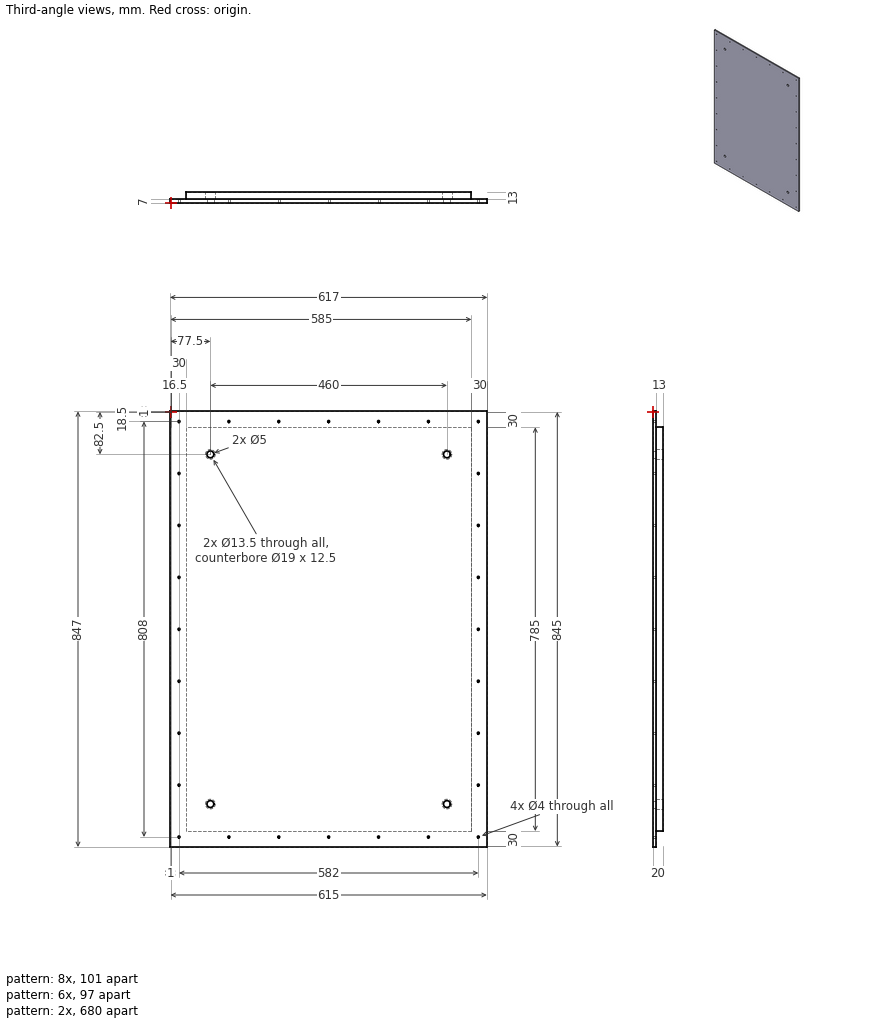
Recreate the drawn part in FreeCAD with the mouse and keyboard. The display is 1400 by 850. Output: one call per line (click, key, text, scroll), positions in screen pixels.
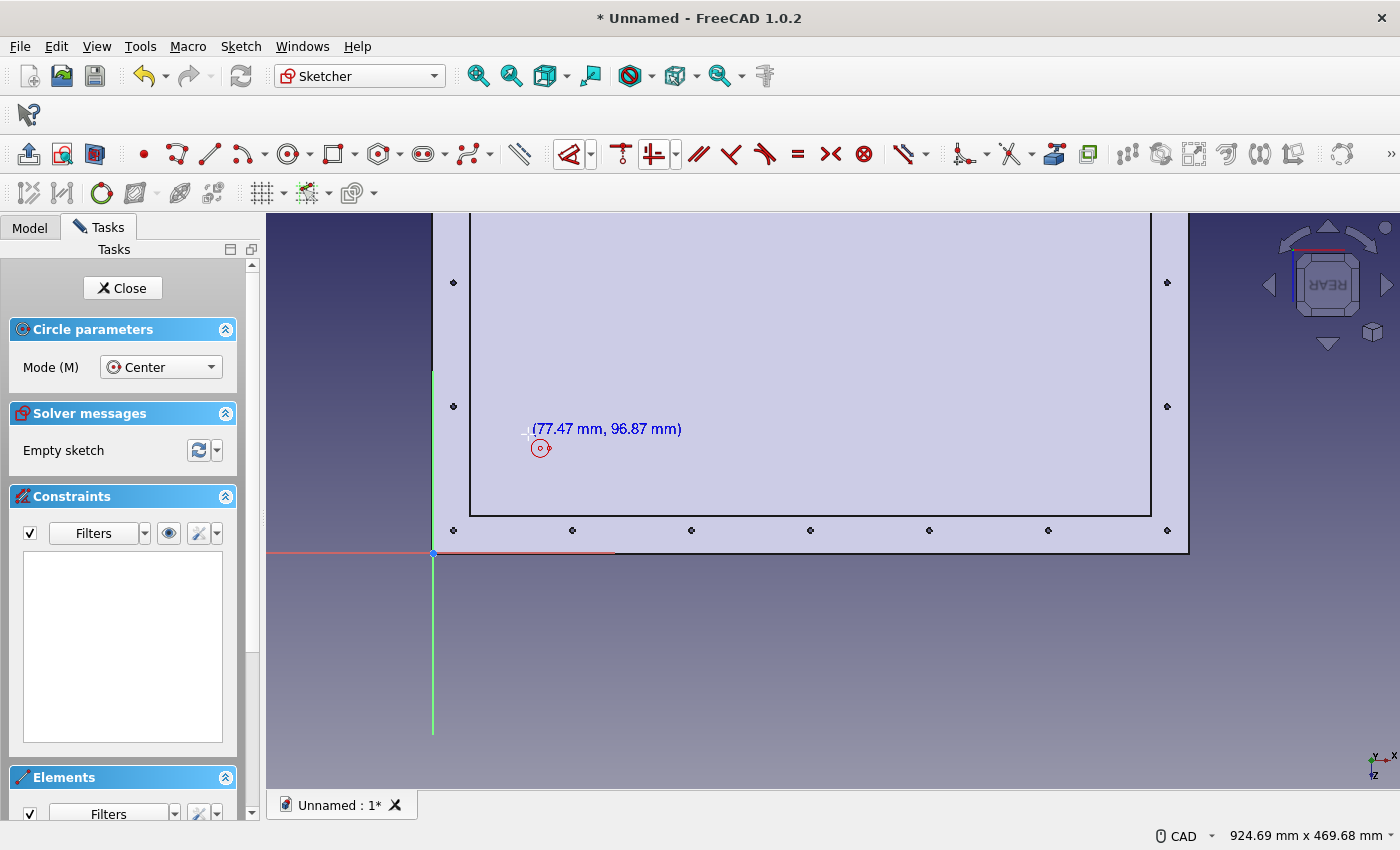
click(528, 452)
move(530, 450)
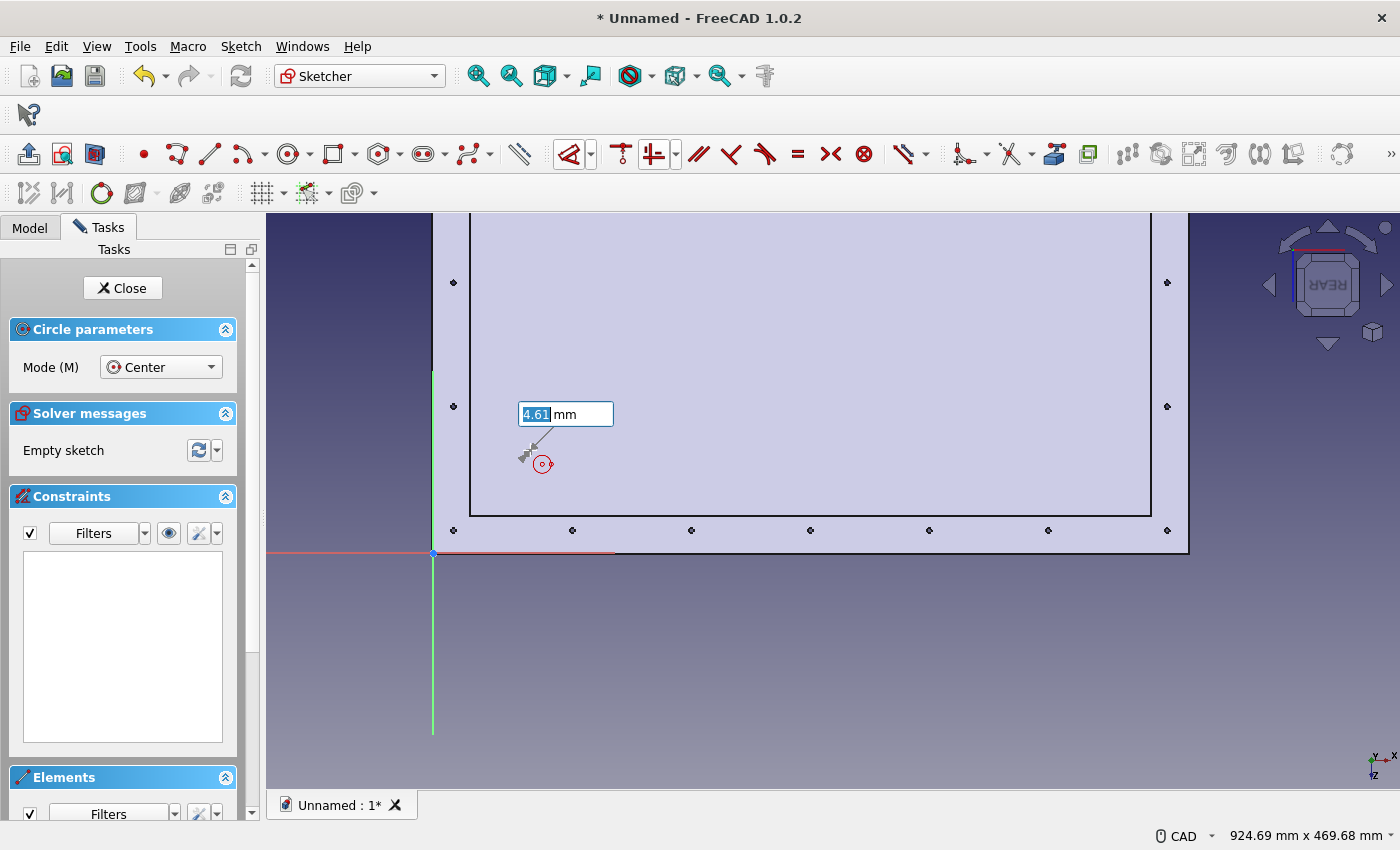
text(5)
key(Return)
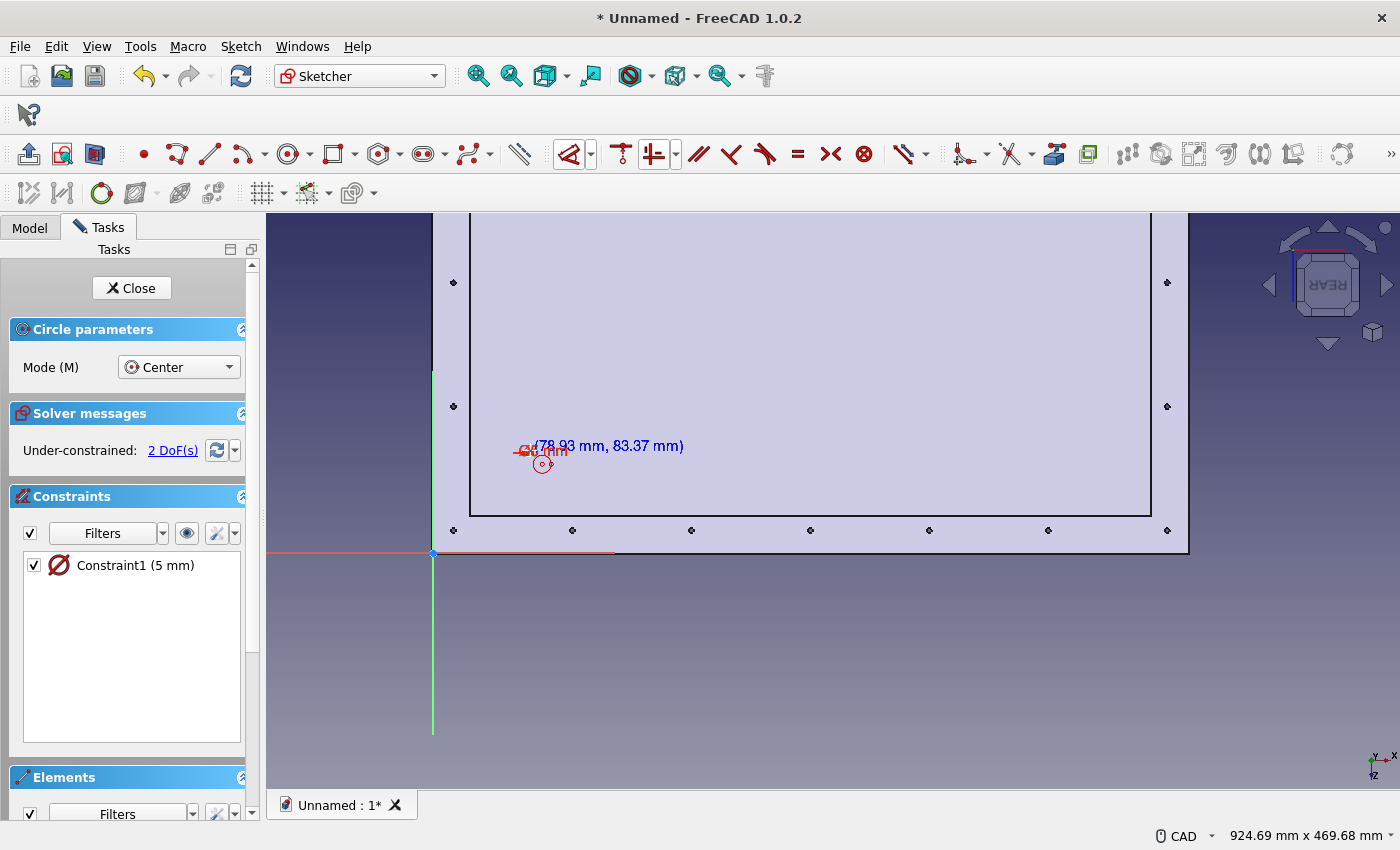
scroll(1092, 452, up, 11)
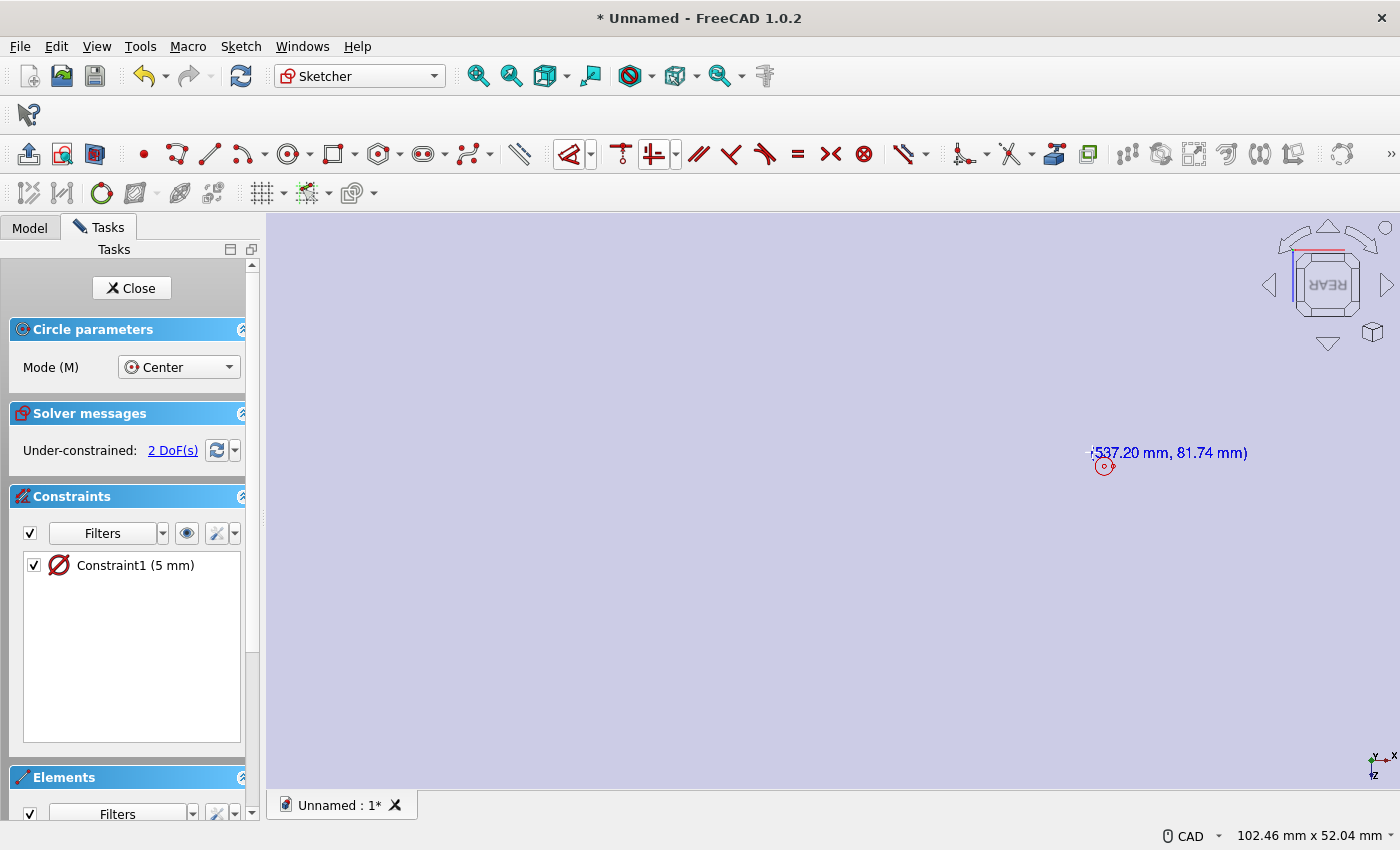
scroll(1093, 452, down, 11)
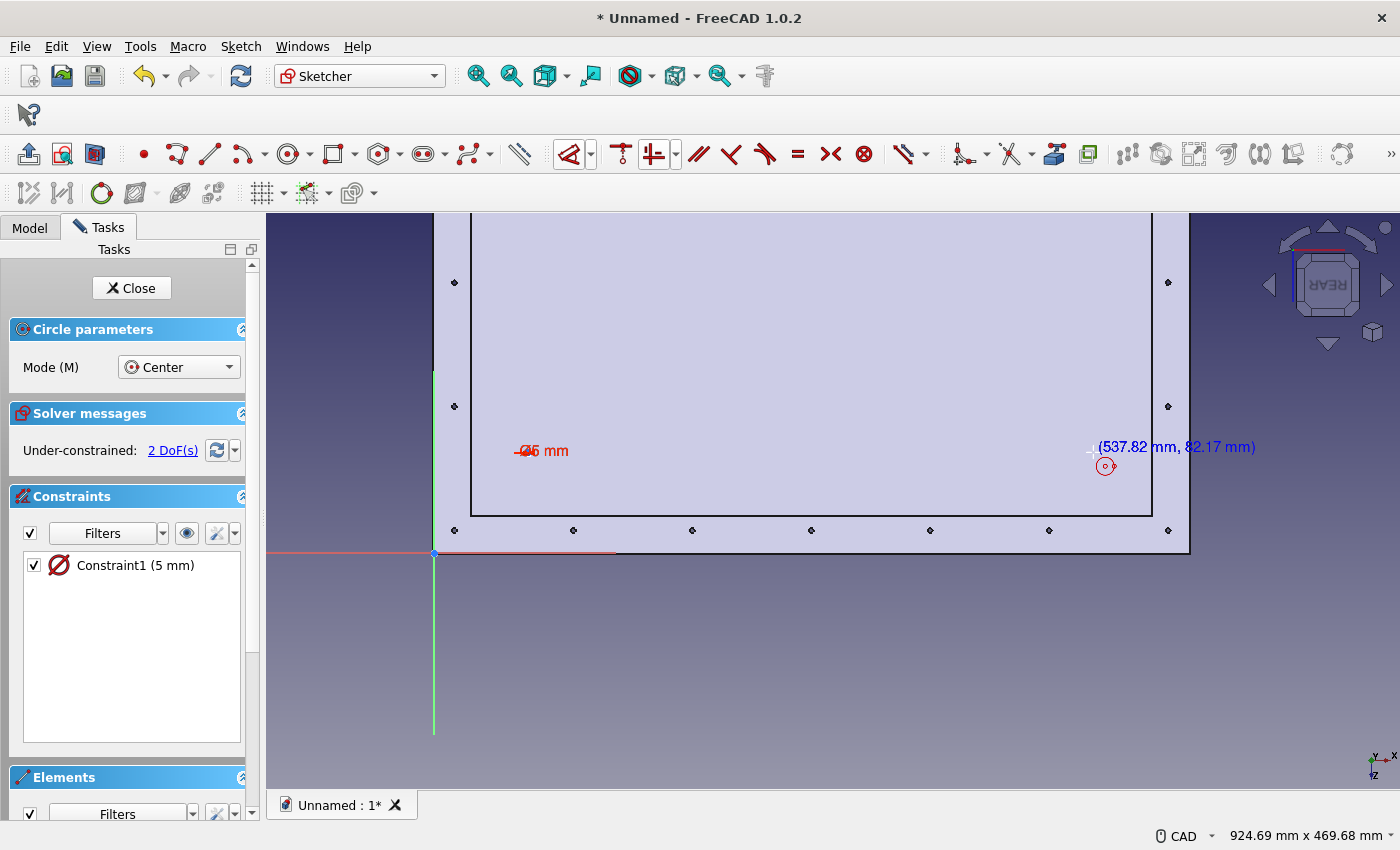
click(1093, 452)
move(1095, 450)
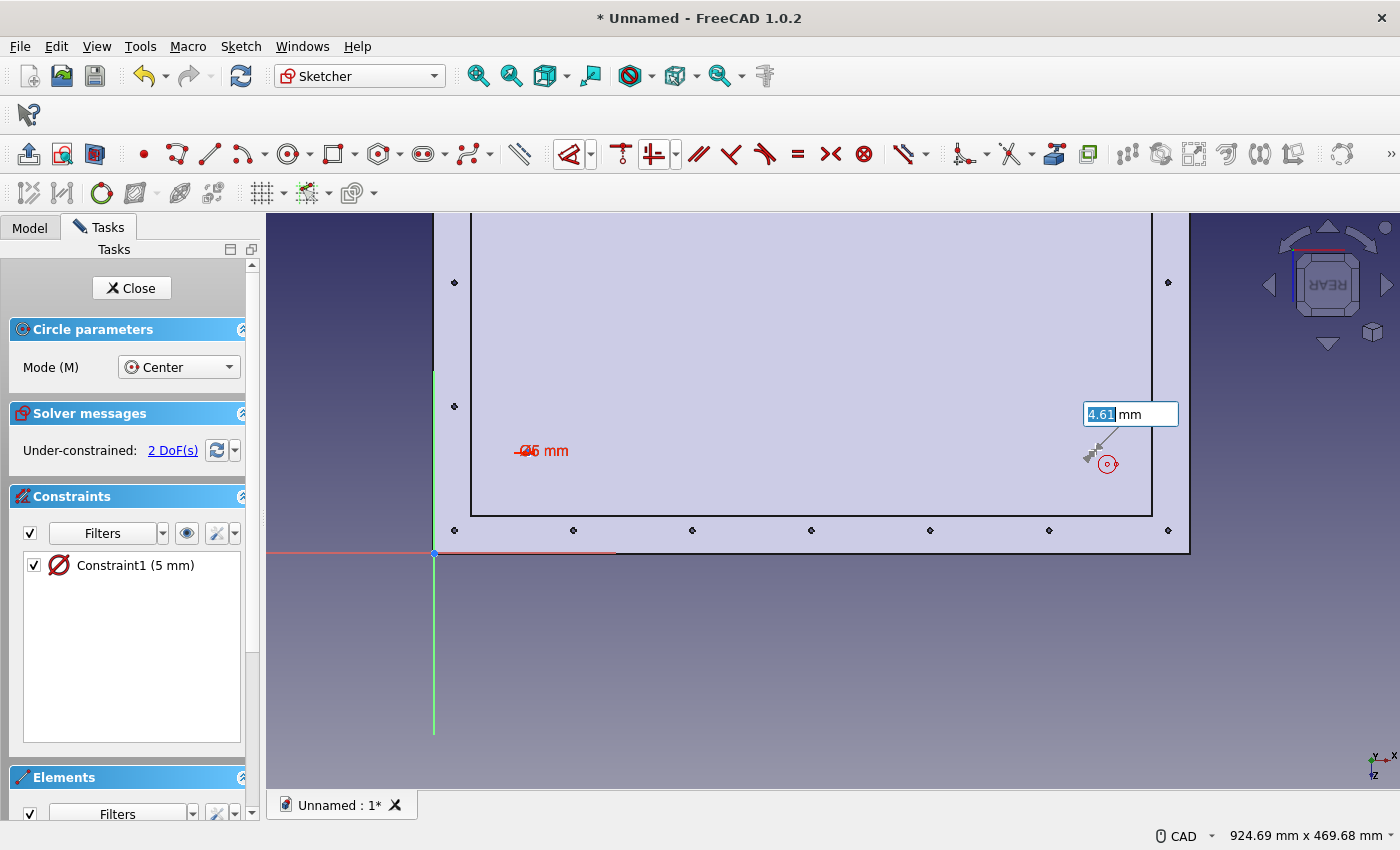
text(5)
key(Return)
key(Escape)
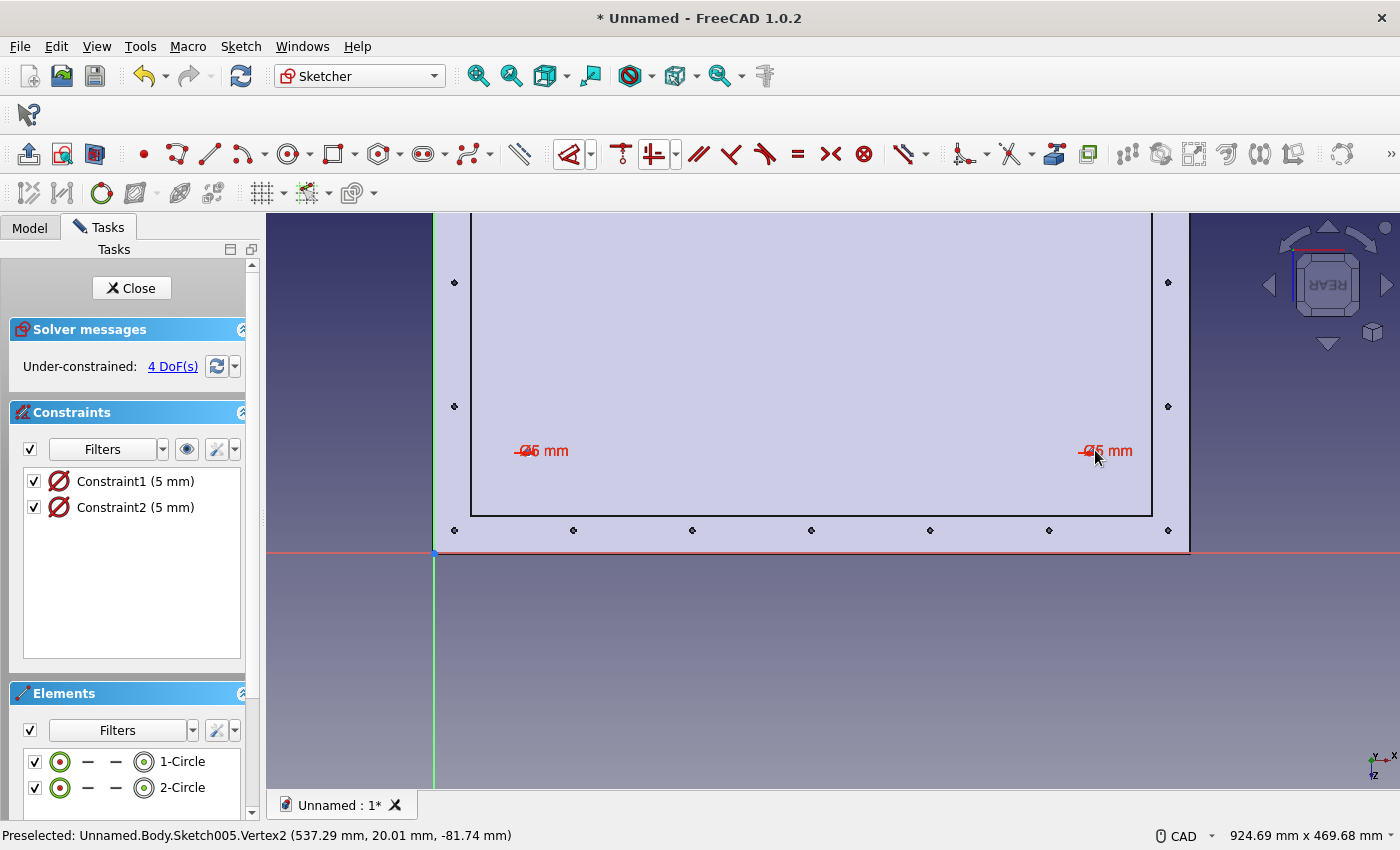
click(529, 453)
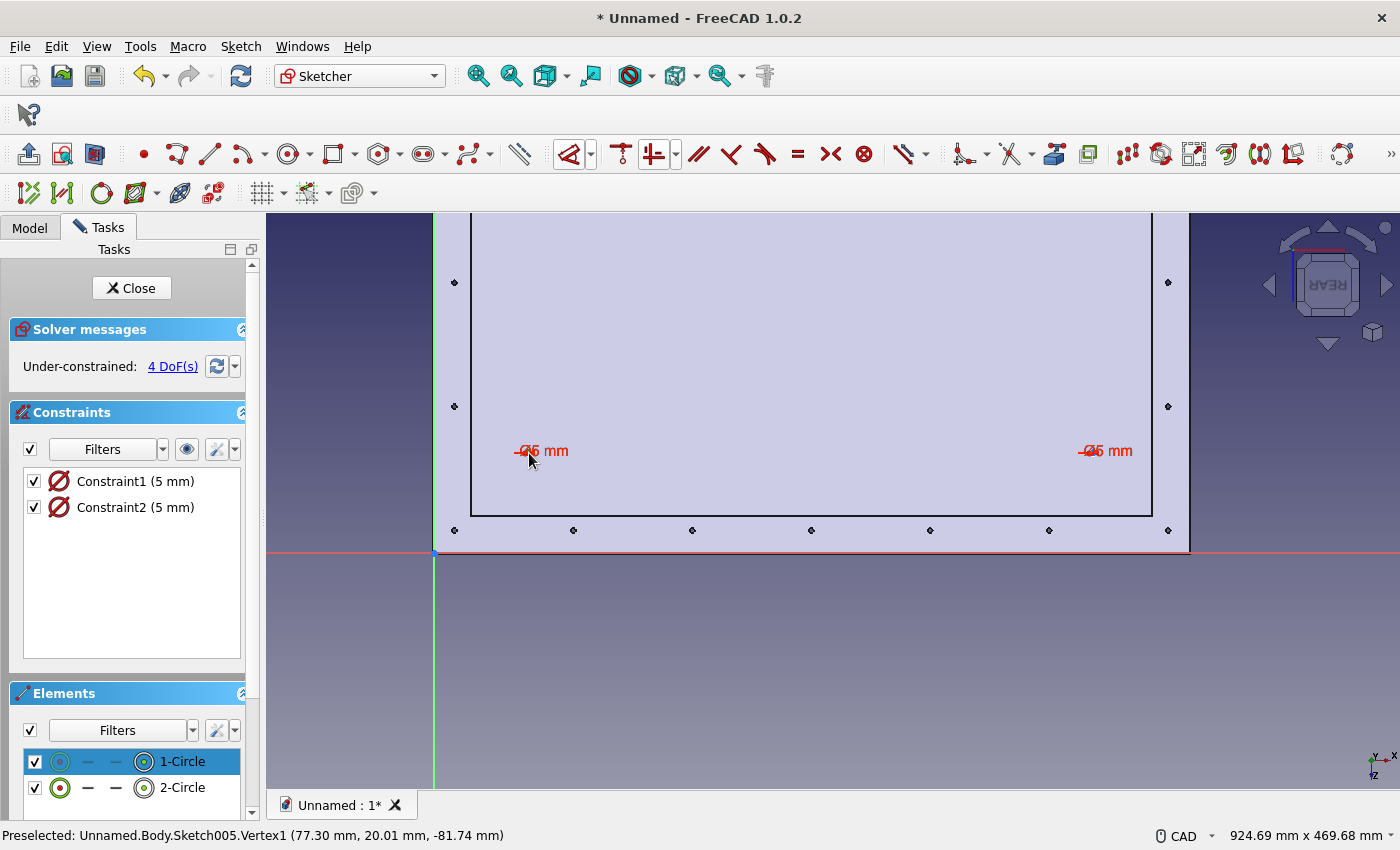
click(1093, 453)